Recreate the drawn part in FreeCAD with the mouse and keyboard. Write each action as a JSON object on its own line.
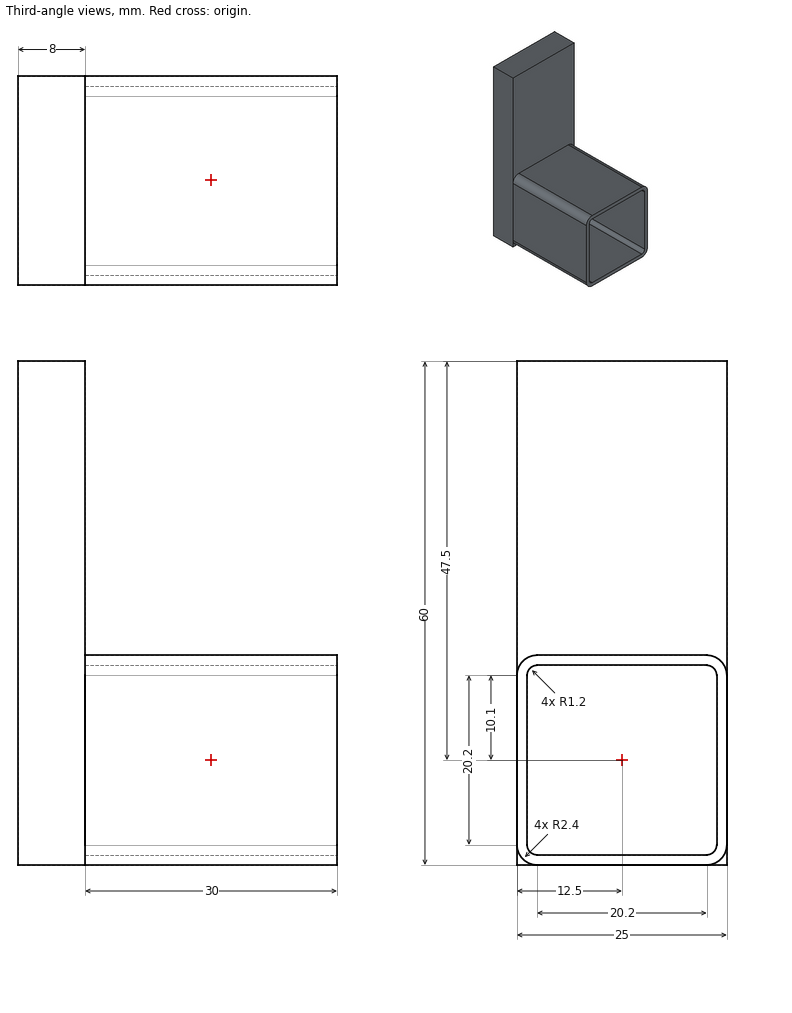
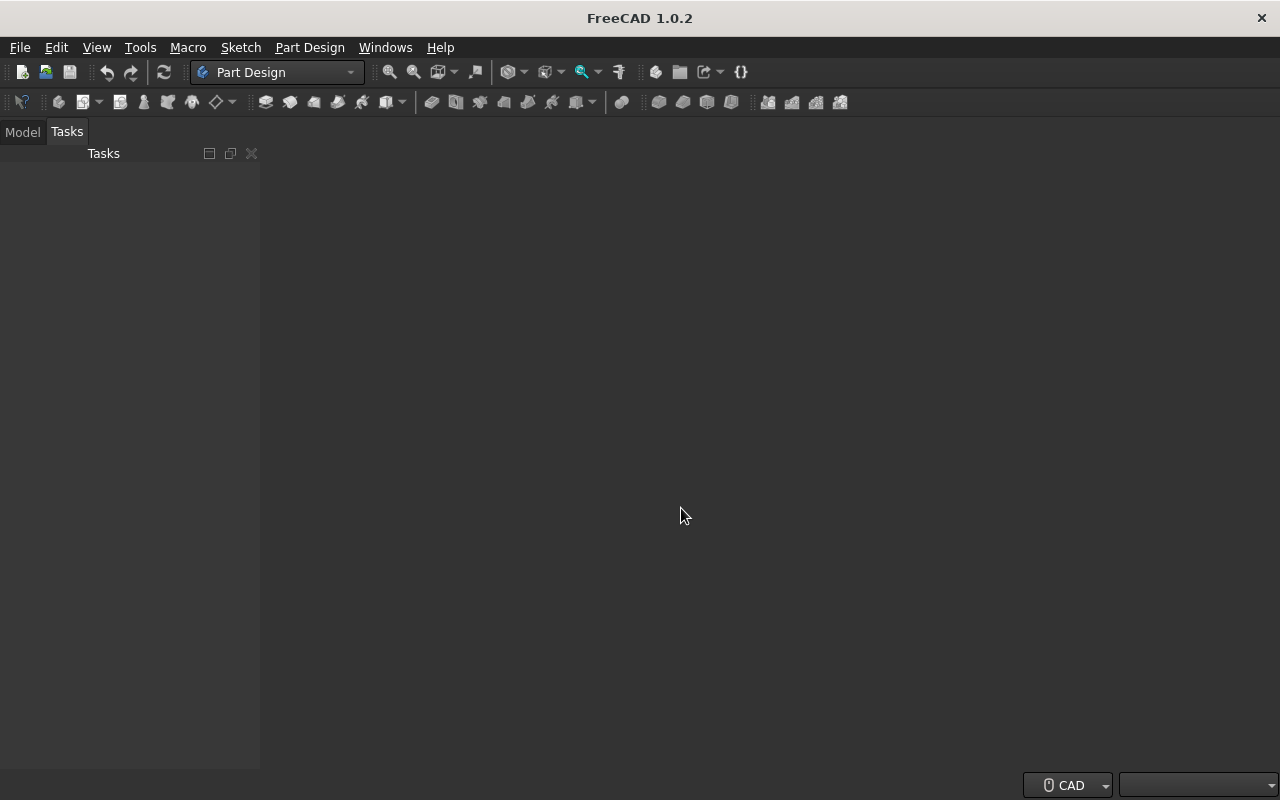
{"action": "key", "text": "ctrl+n"}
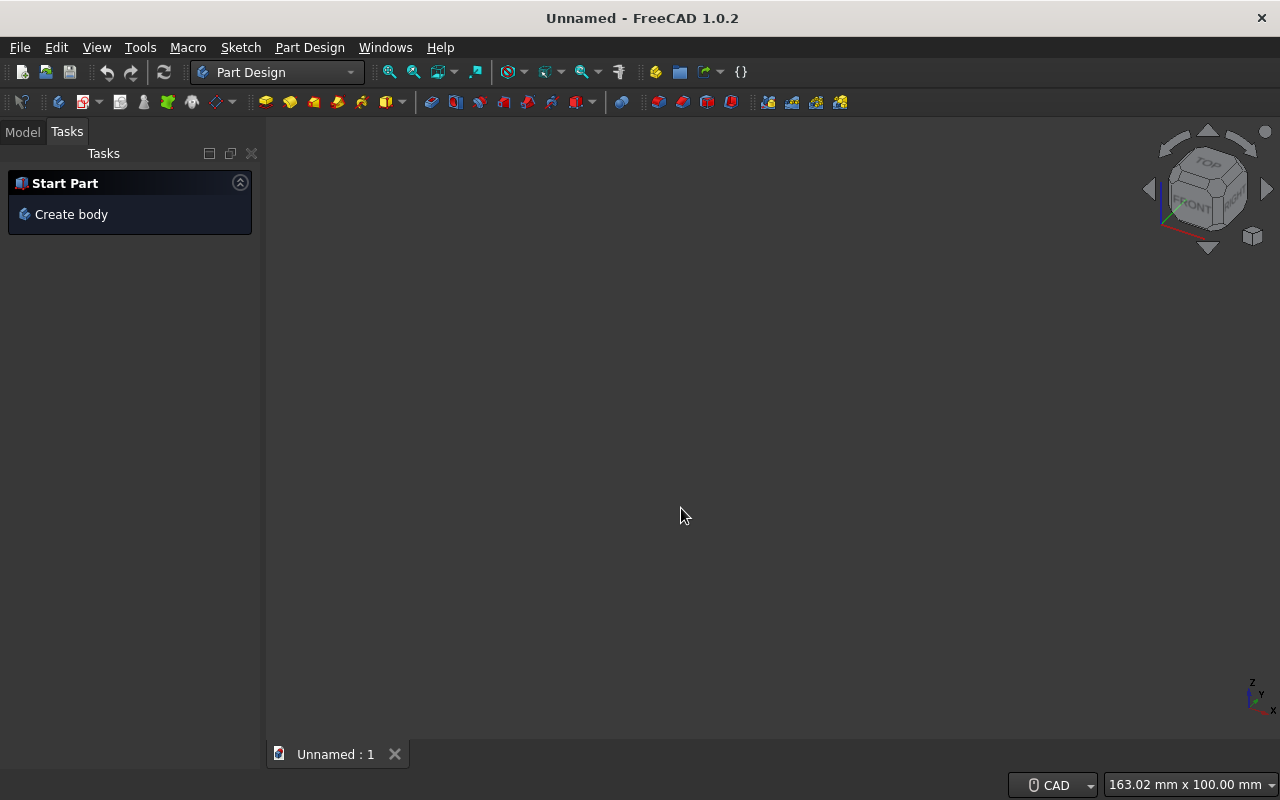
{"action": "left_click", "coordinate": [60, 102]}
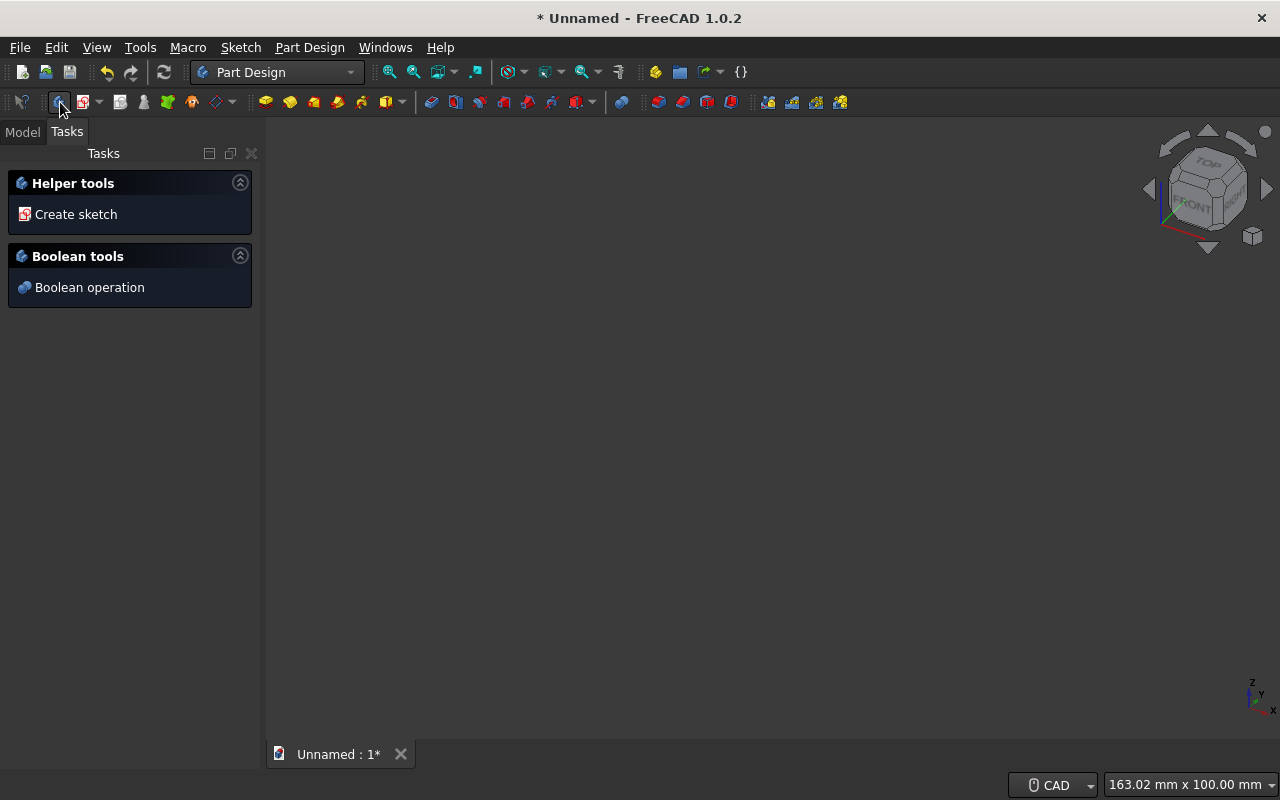
{"action": "left_click", "coordinate": [23, 131]}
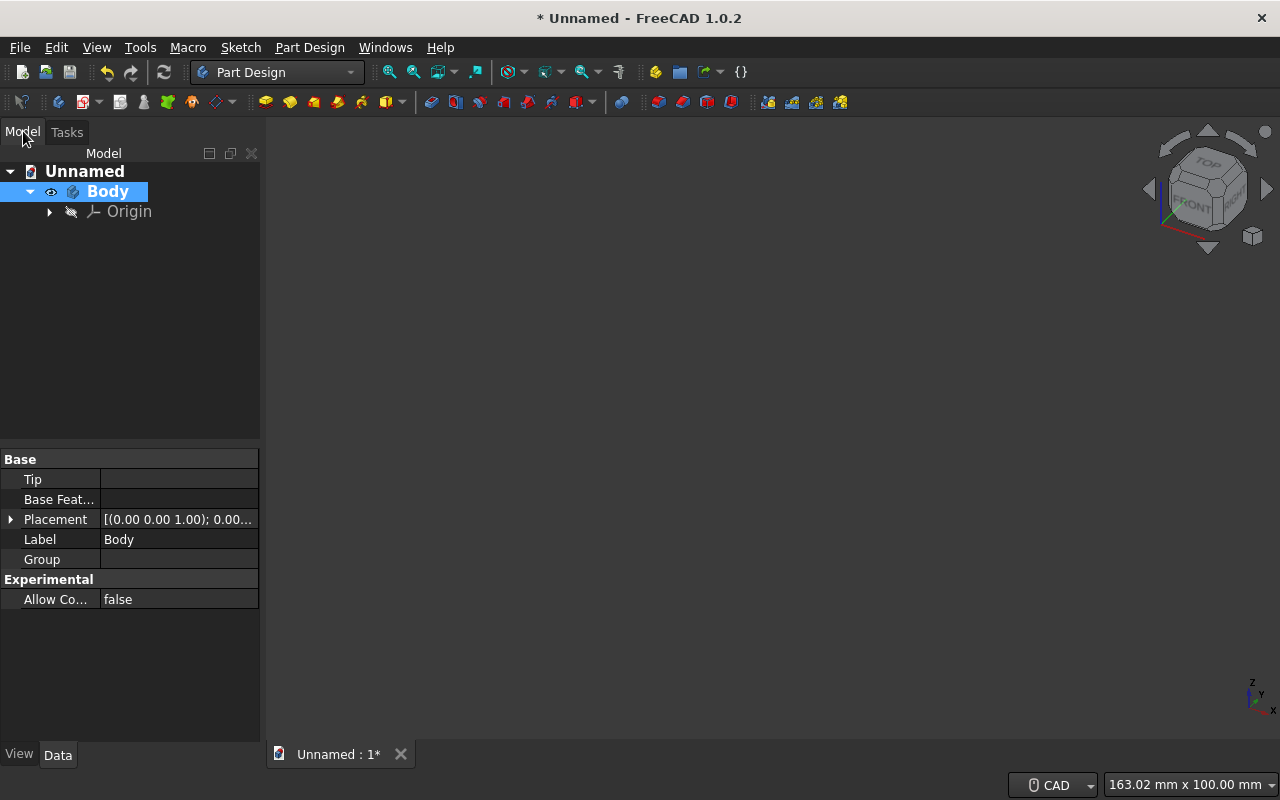
{"action": "left_click", "coordinate": [50, 212]}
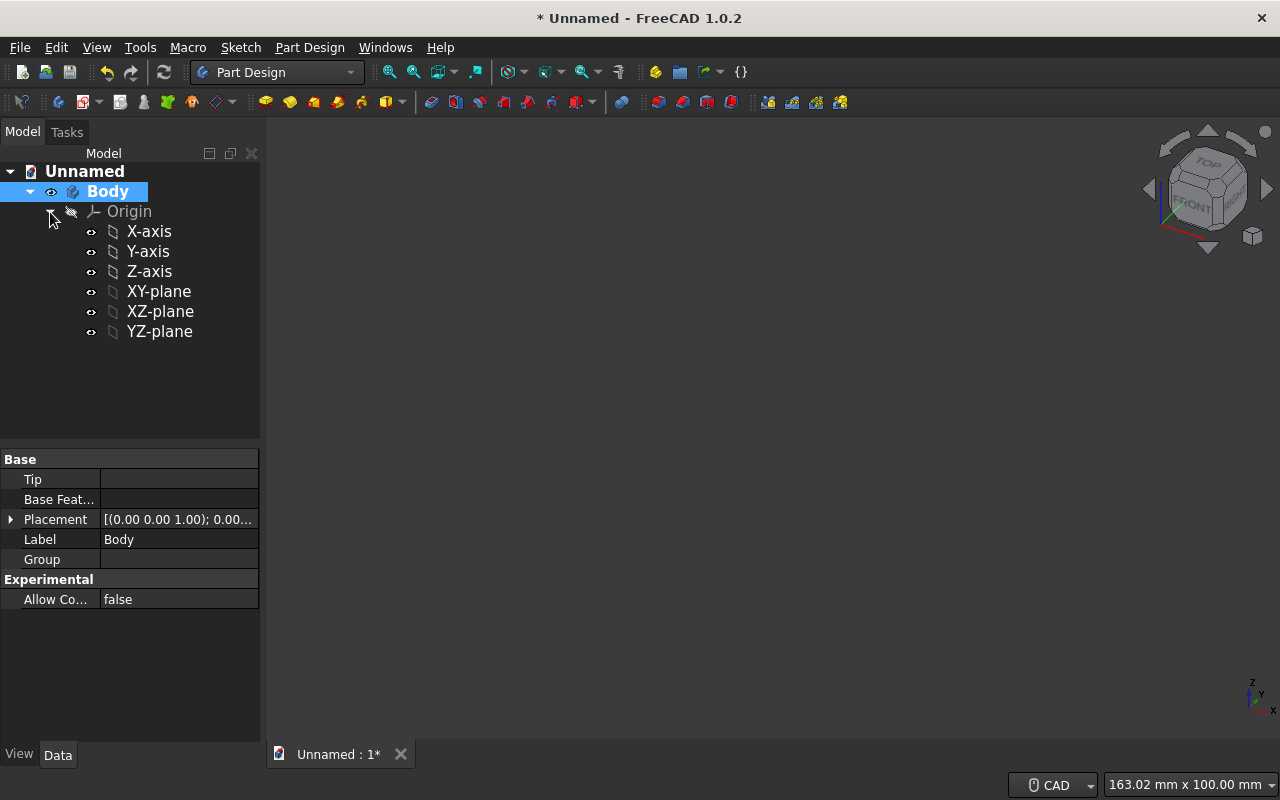
{"action": "left_click", "coordinate": [136, 332]}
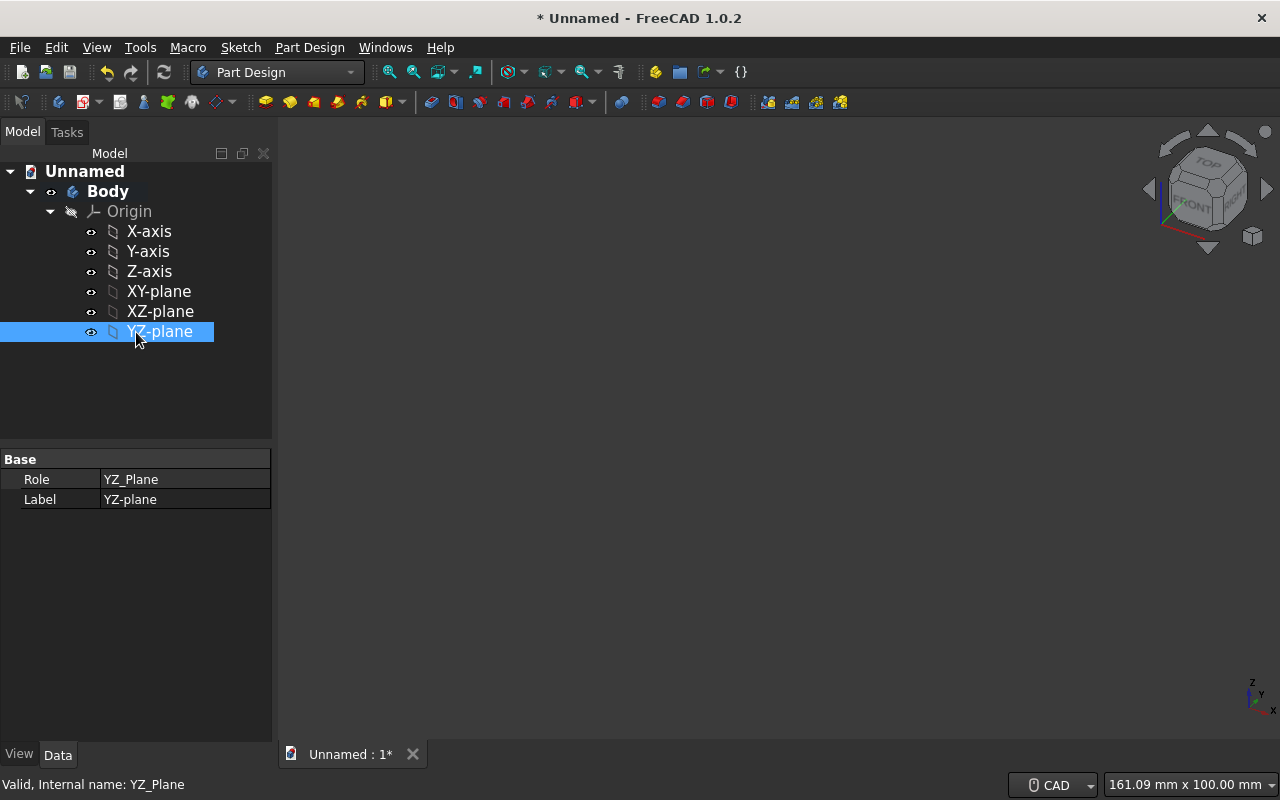
{"action": "left_click", "coordinate": [216, 102]}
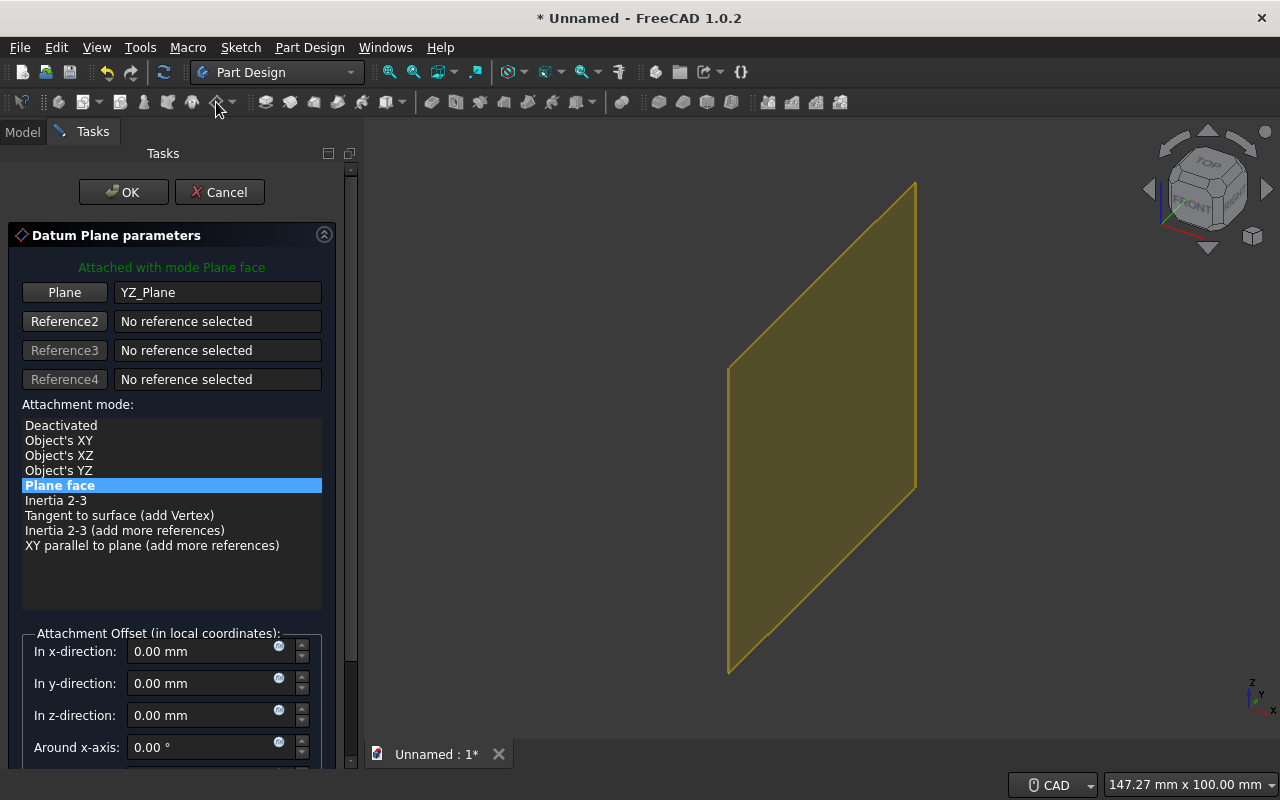
{"action": "triple_click", "coordinate": [210, 715]}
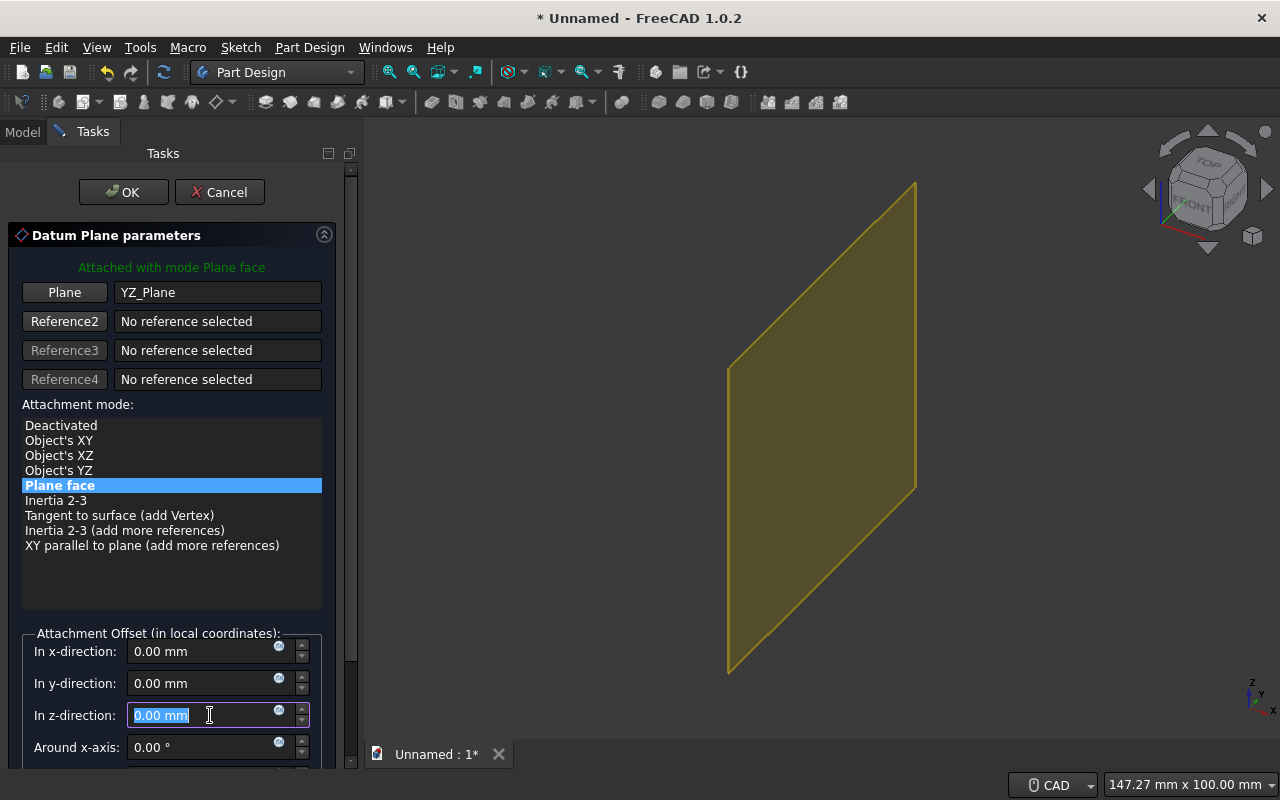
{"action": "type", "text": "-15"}
{"action": "key", "text": "Tab"}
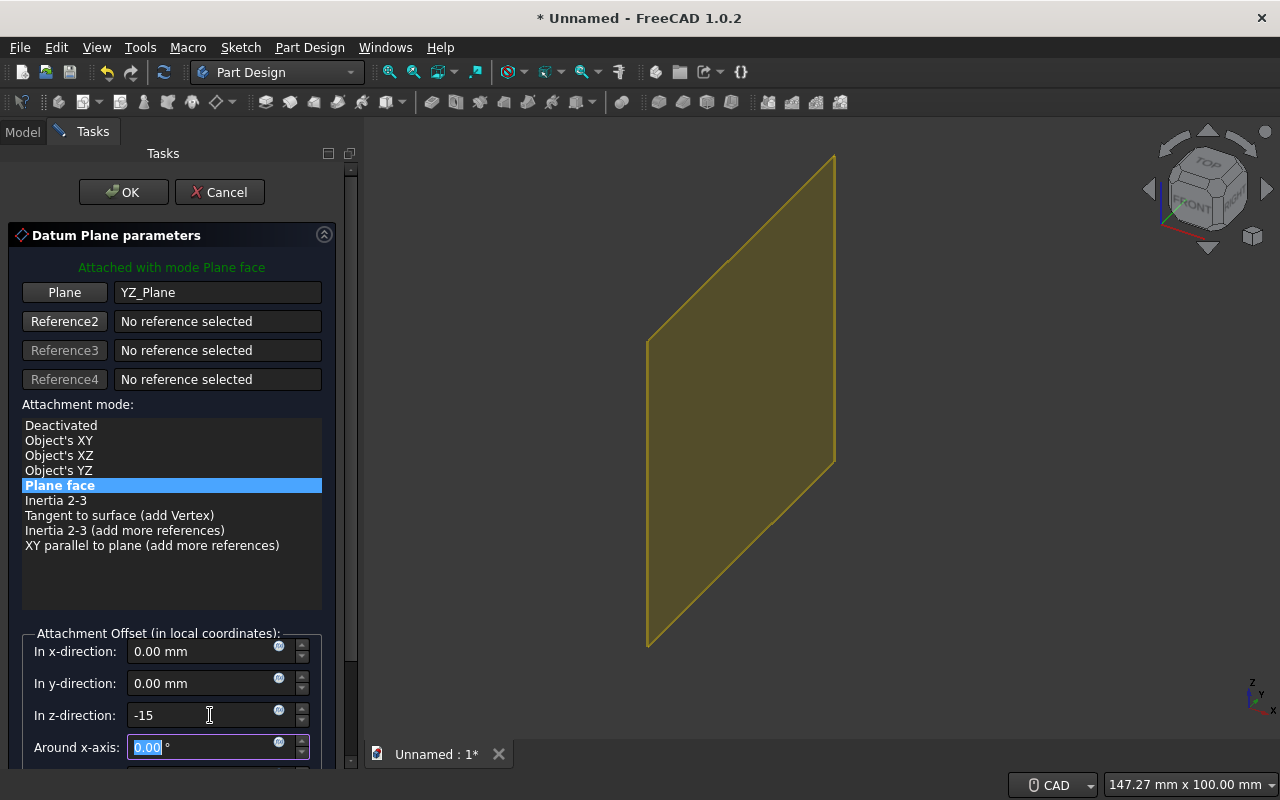
{"action": "left_click", "coordinate": [124, 192]}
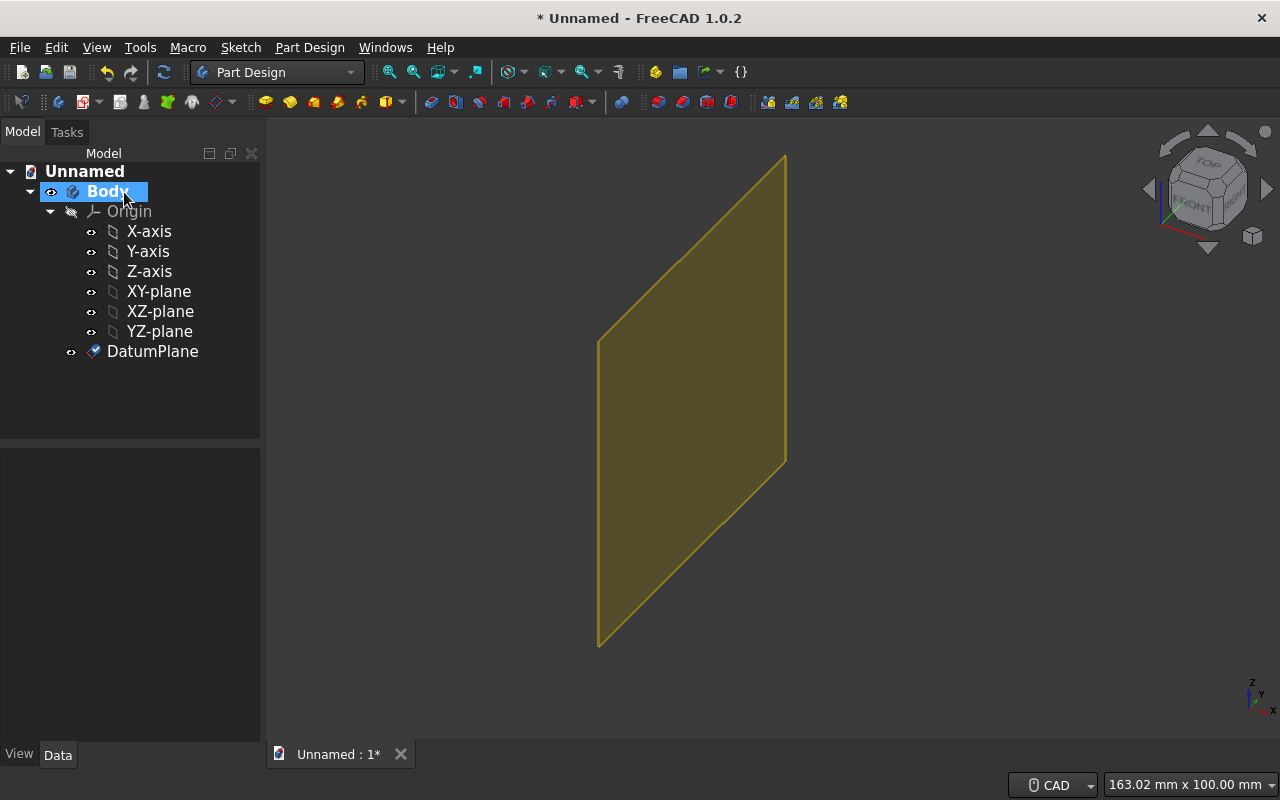
{"action": "left_click", "coordinate": [116, 352]}